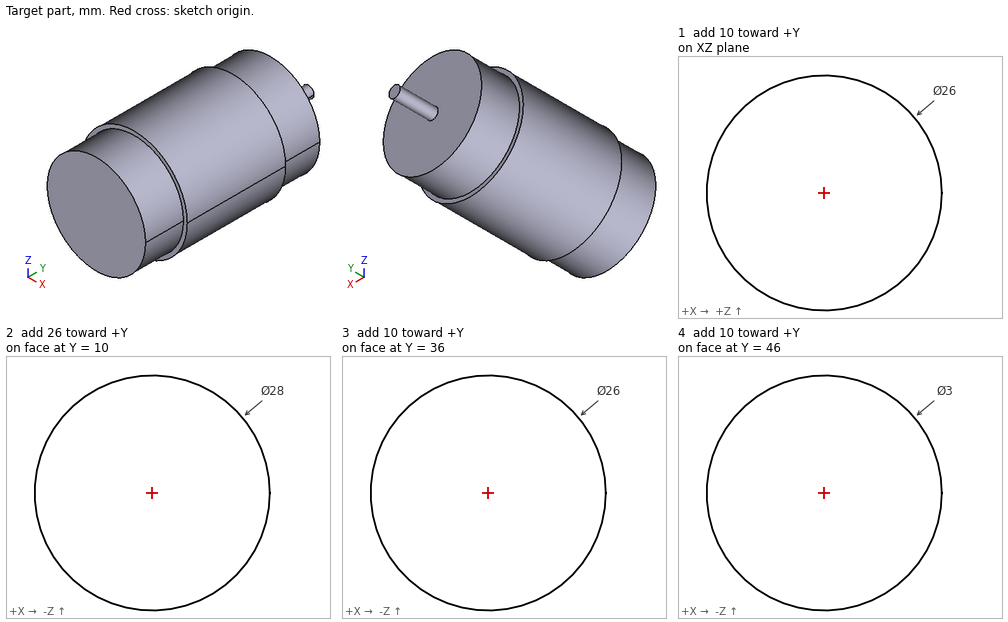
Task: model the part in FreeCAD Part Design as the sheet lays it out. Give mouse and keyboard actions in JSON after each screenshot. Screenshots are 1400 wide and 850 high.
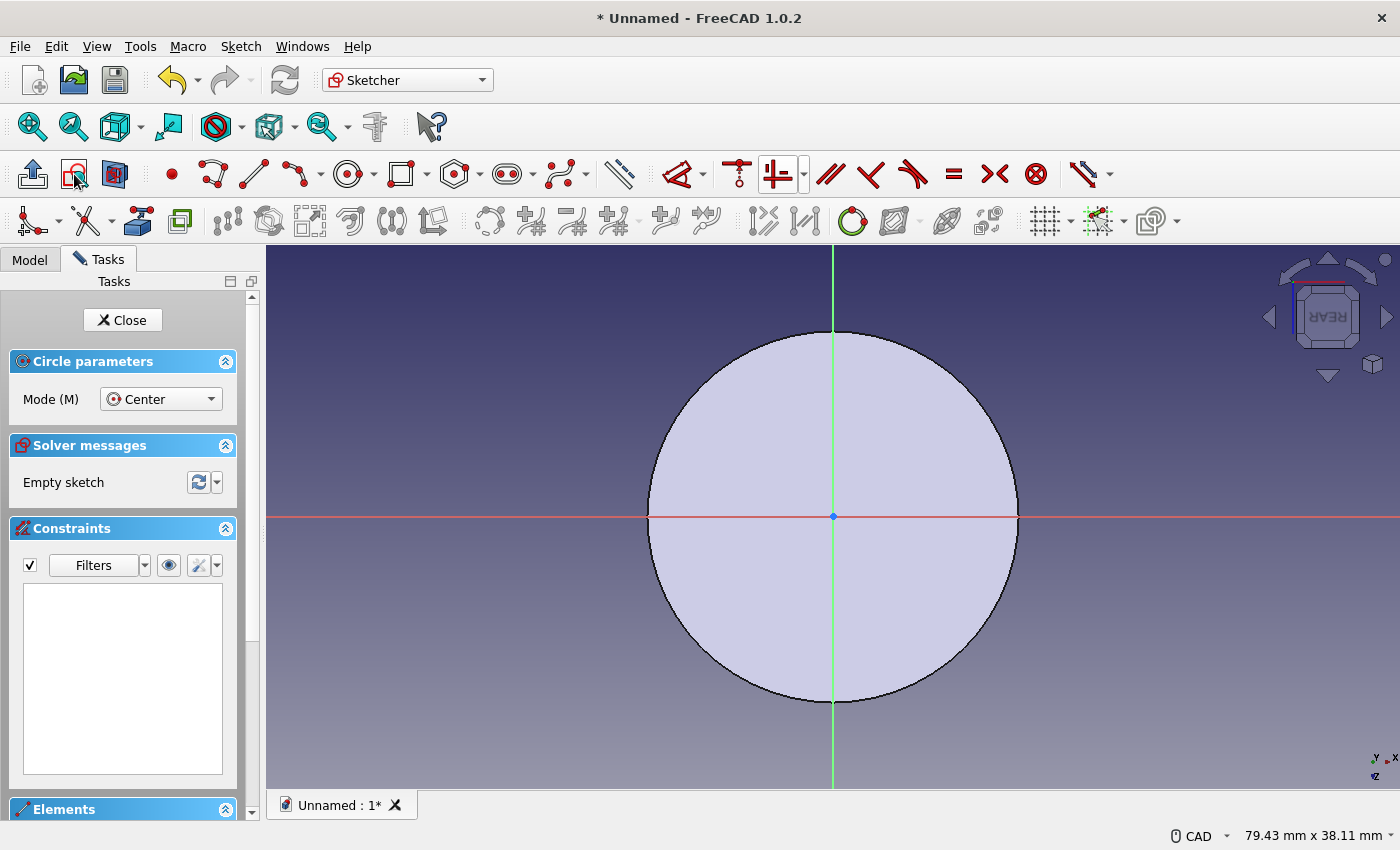
{"action": "left_click", "coordinate": [833, 517]}
{"action": "mouse_move", "coordinate": [974, 376]}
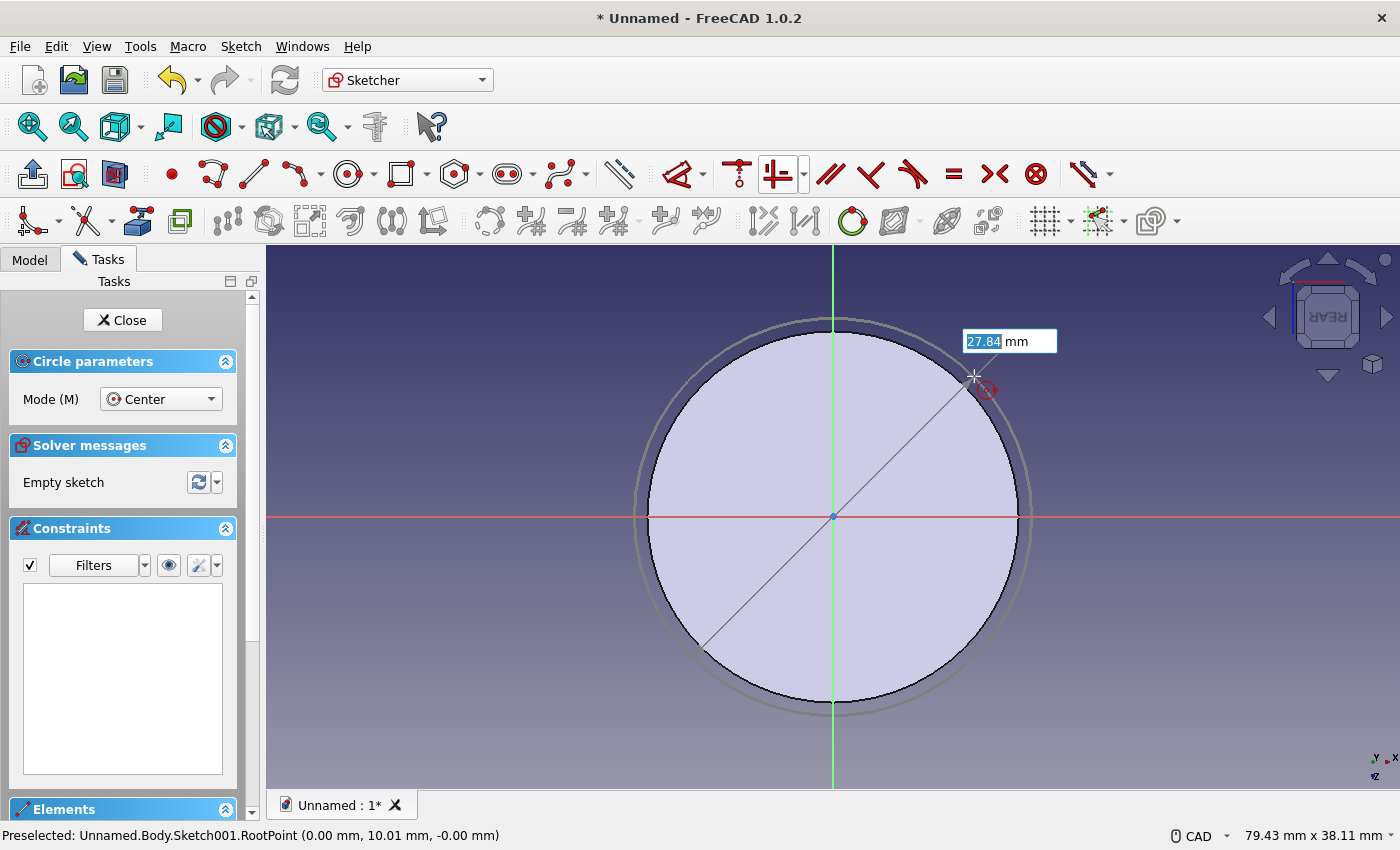
{"action": "type", "text": "28"}
{"action": "key", "text": "Return"}
{"action": "key", "text": "Escape"}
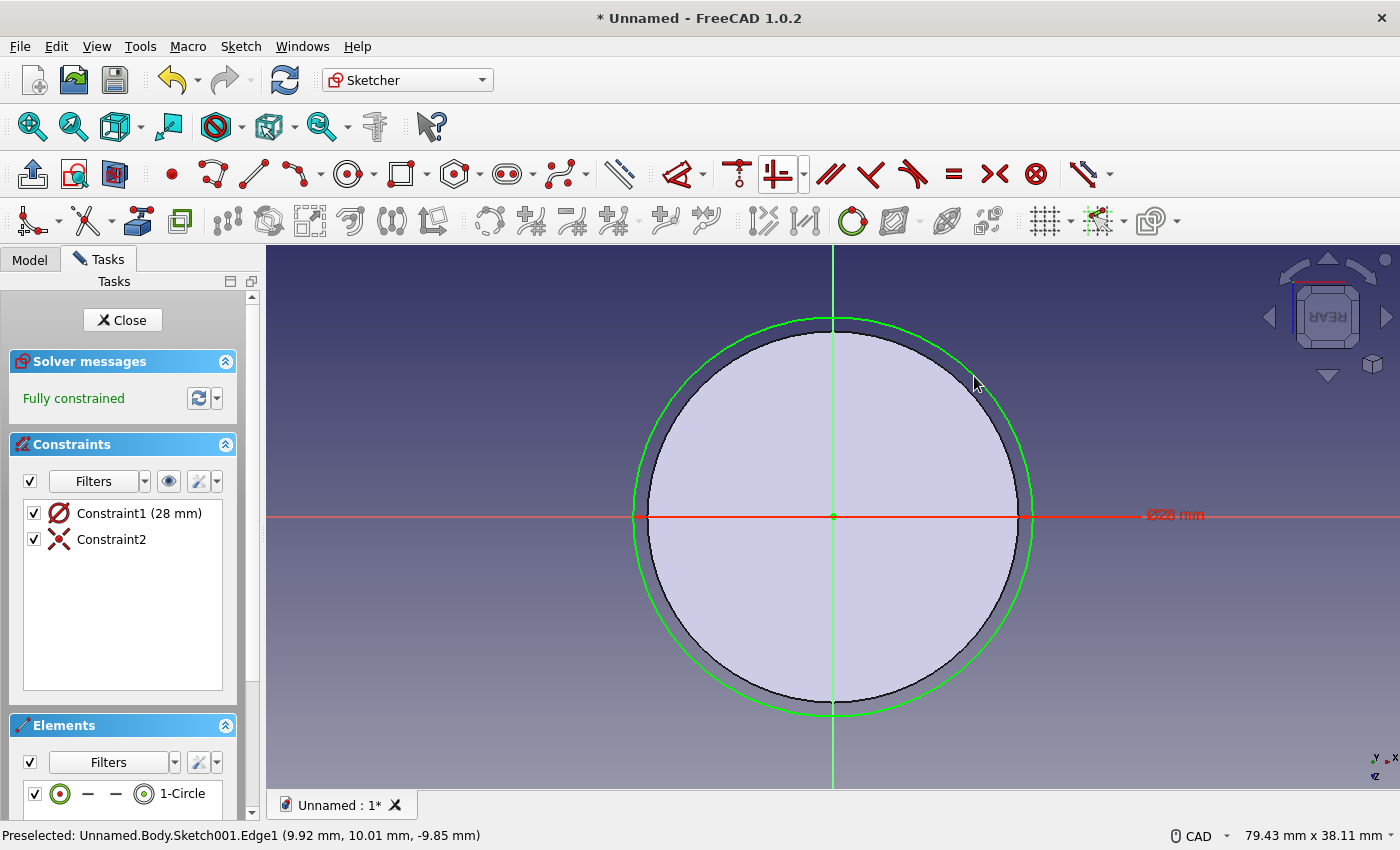
{"action": "left_click", "coordinate": [123, 320]}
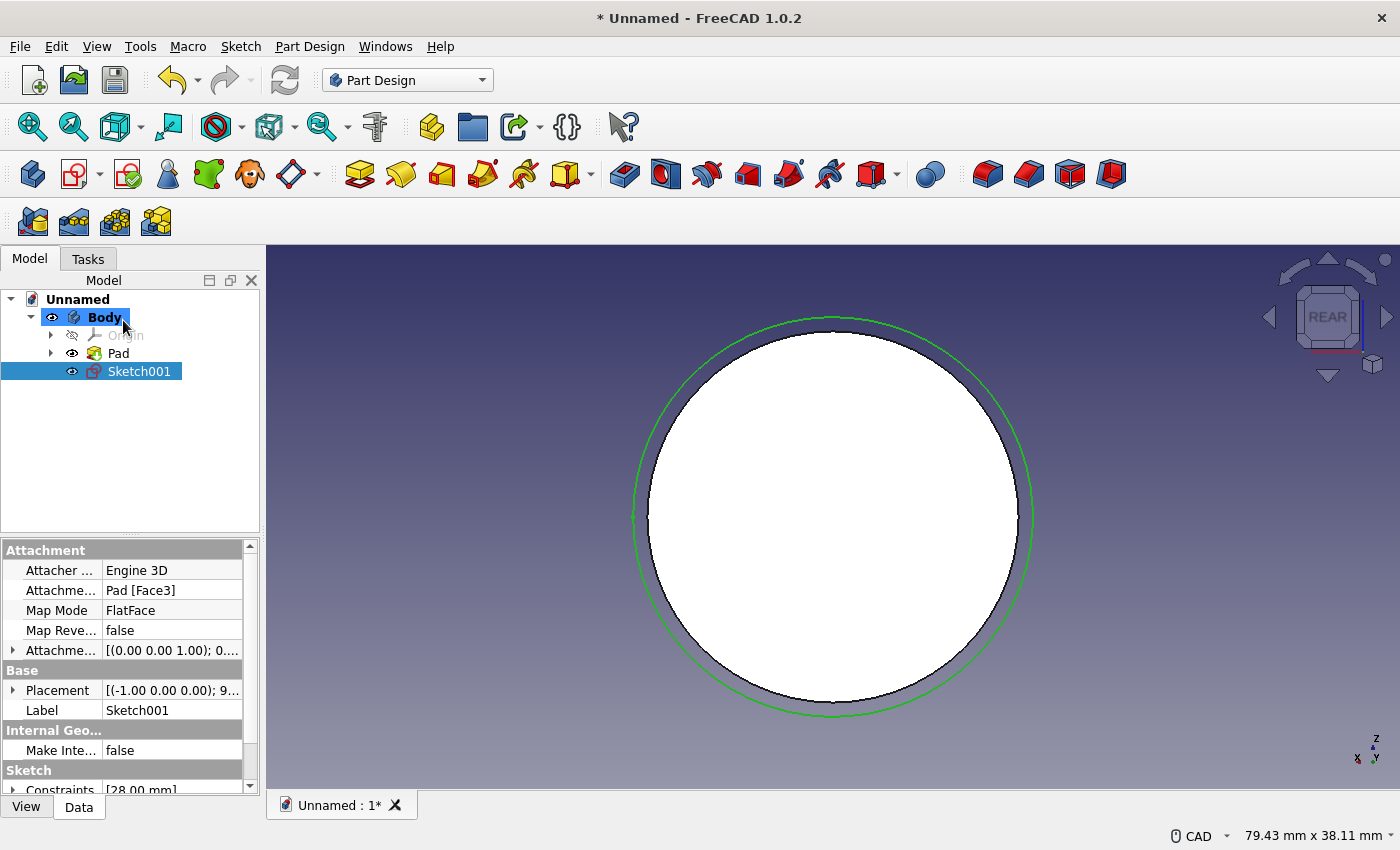
{"action": "left_click", "coordinate": [360, 174]}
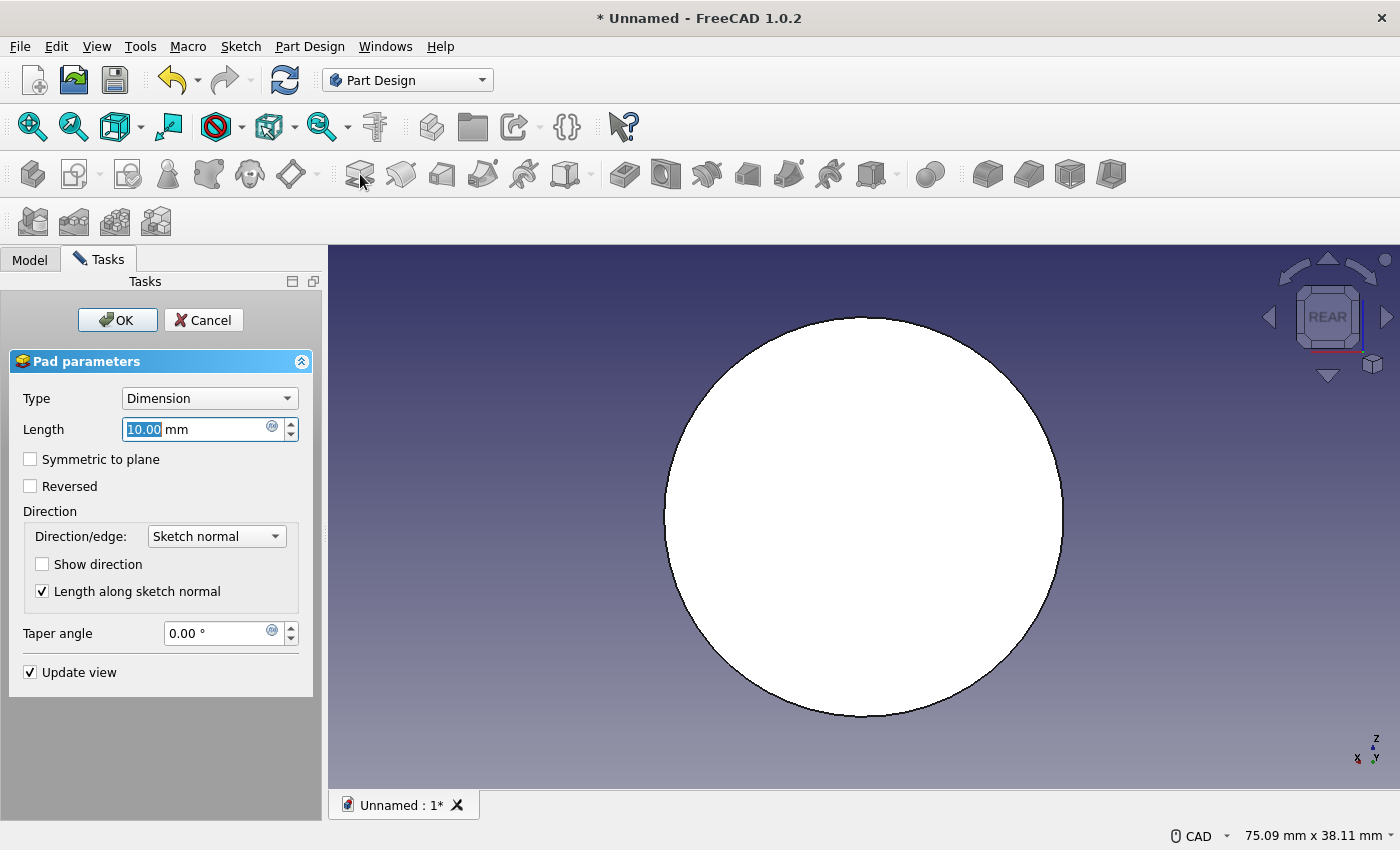
{"action": "type", "text": "26"}
{"action": "key", "text": "Tab"}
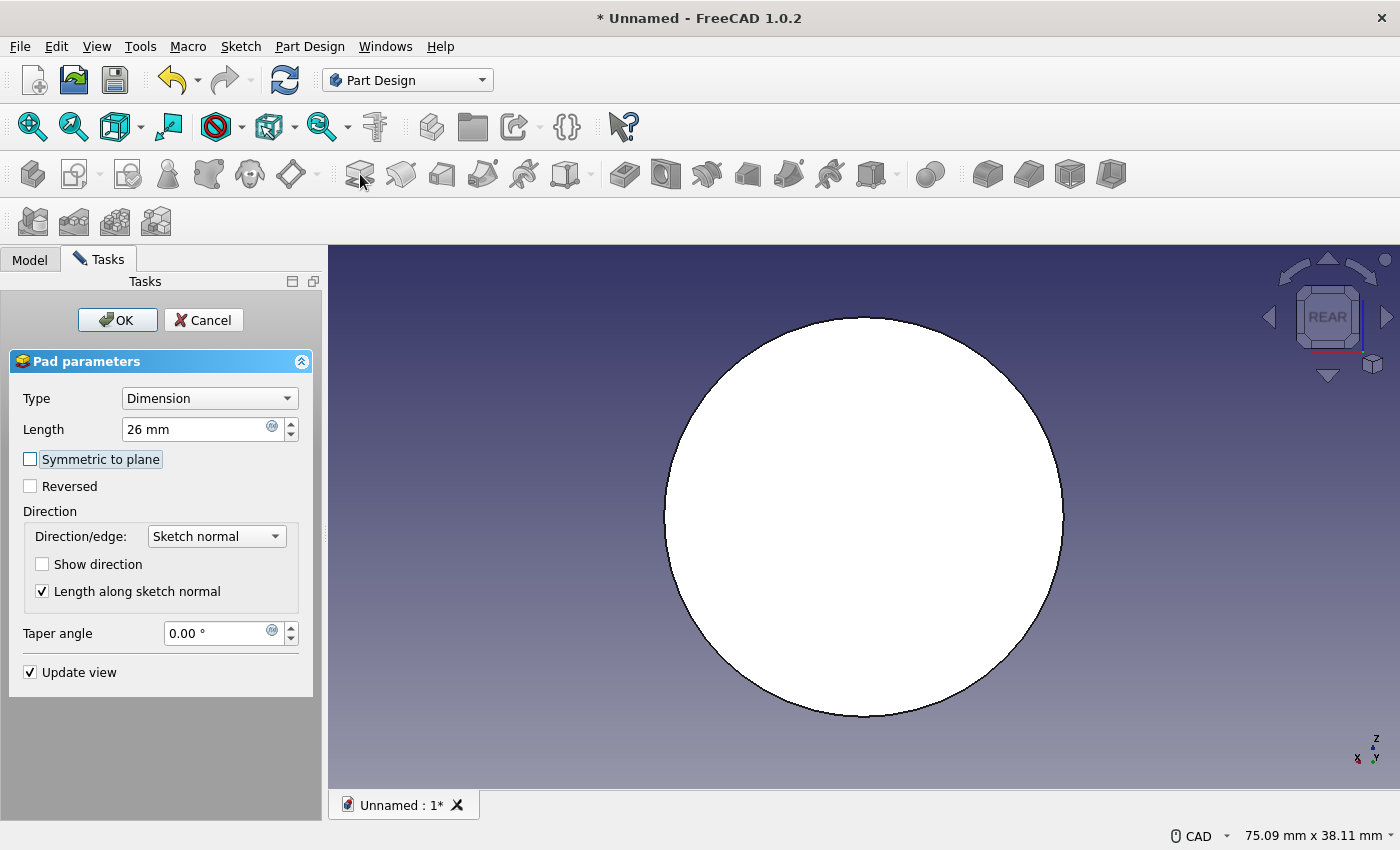
{"action": "left_click", "coordinate": [118, 320]}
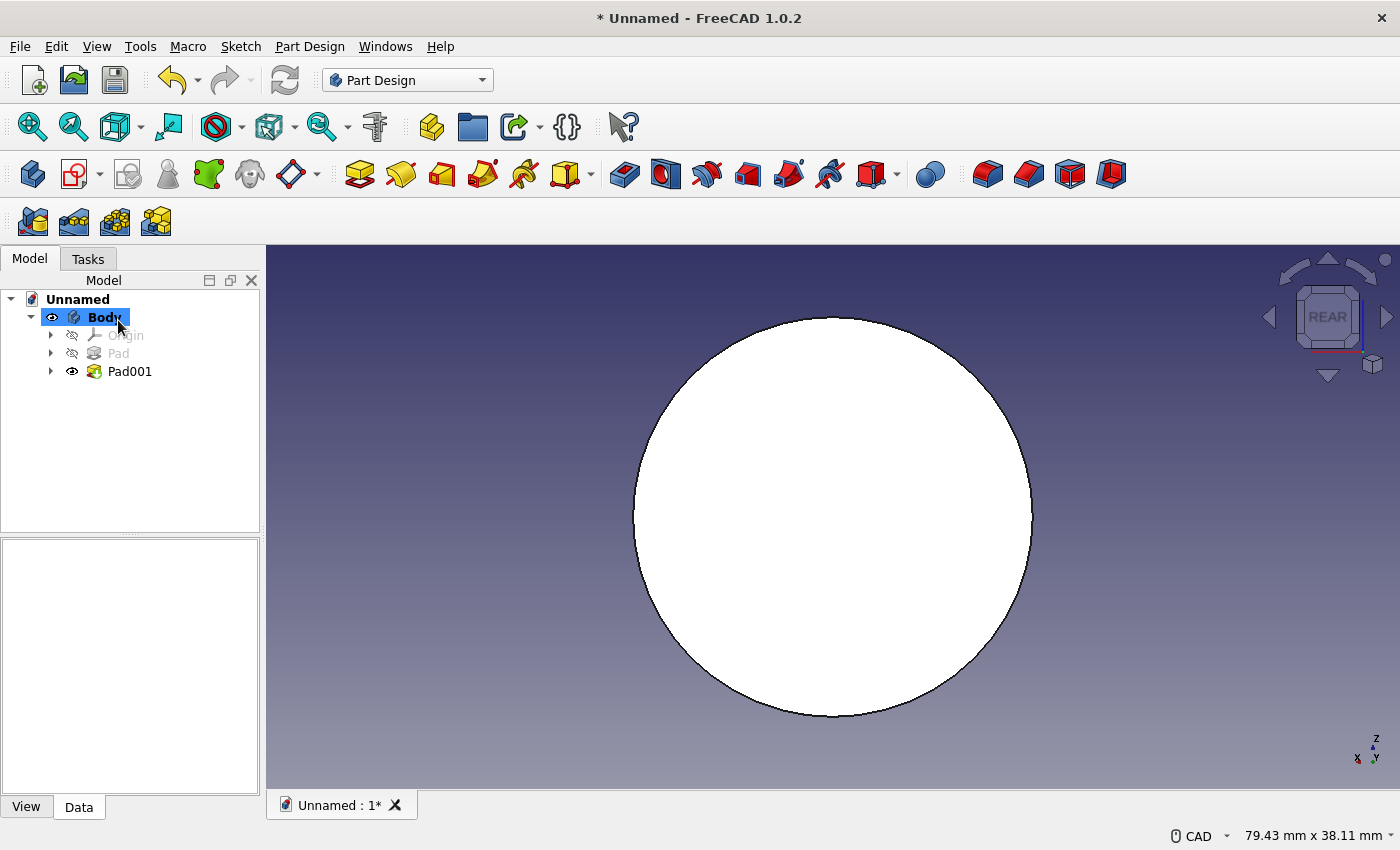
{"action": "left_click", "coordinate": [833, 516]}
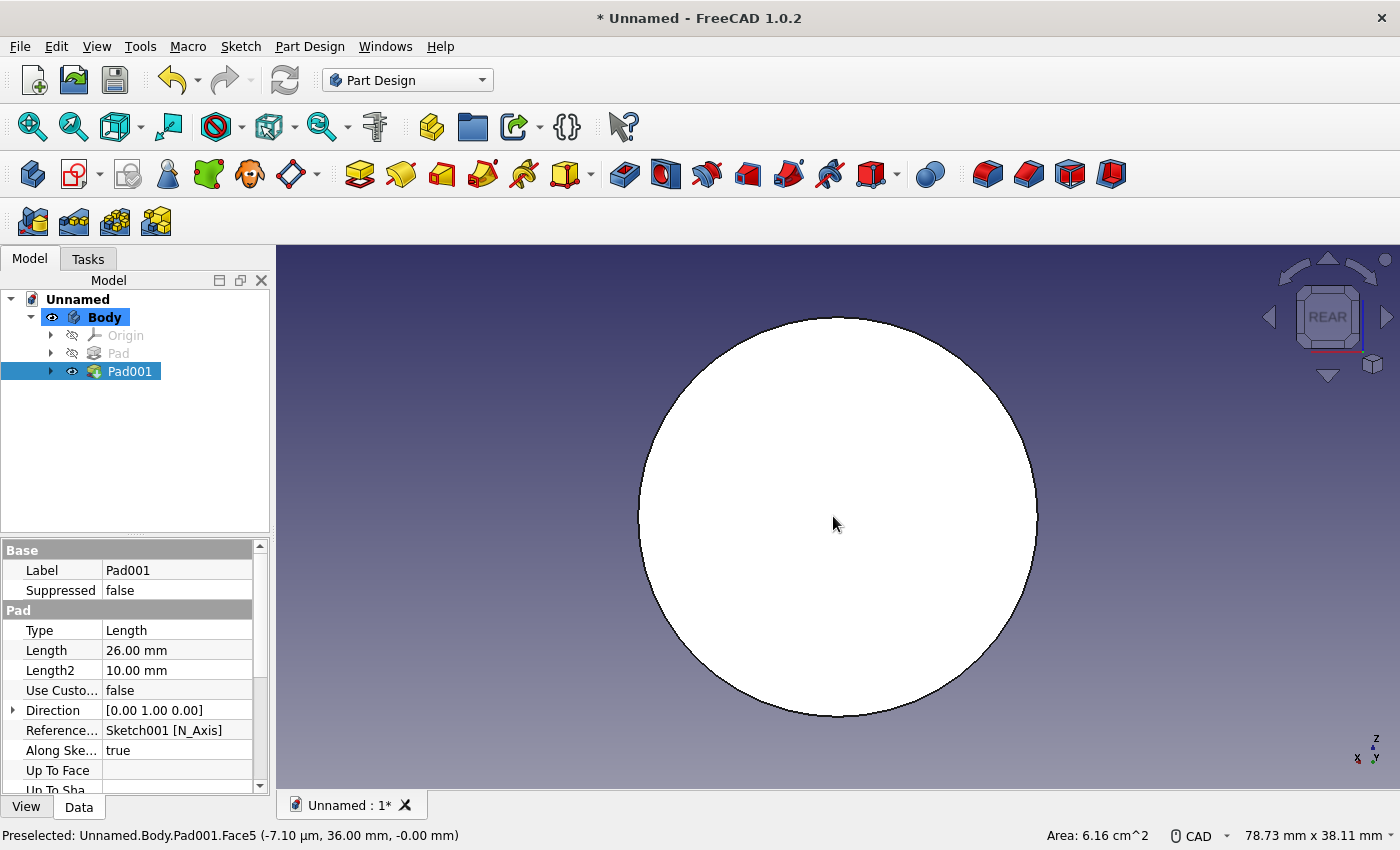
{"action": "left_click", "coordinate": [74, 174]}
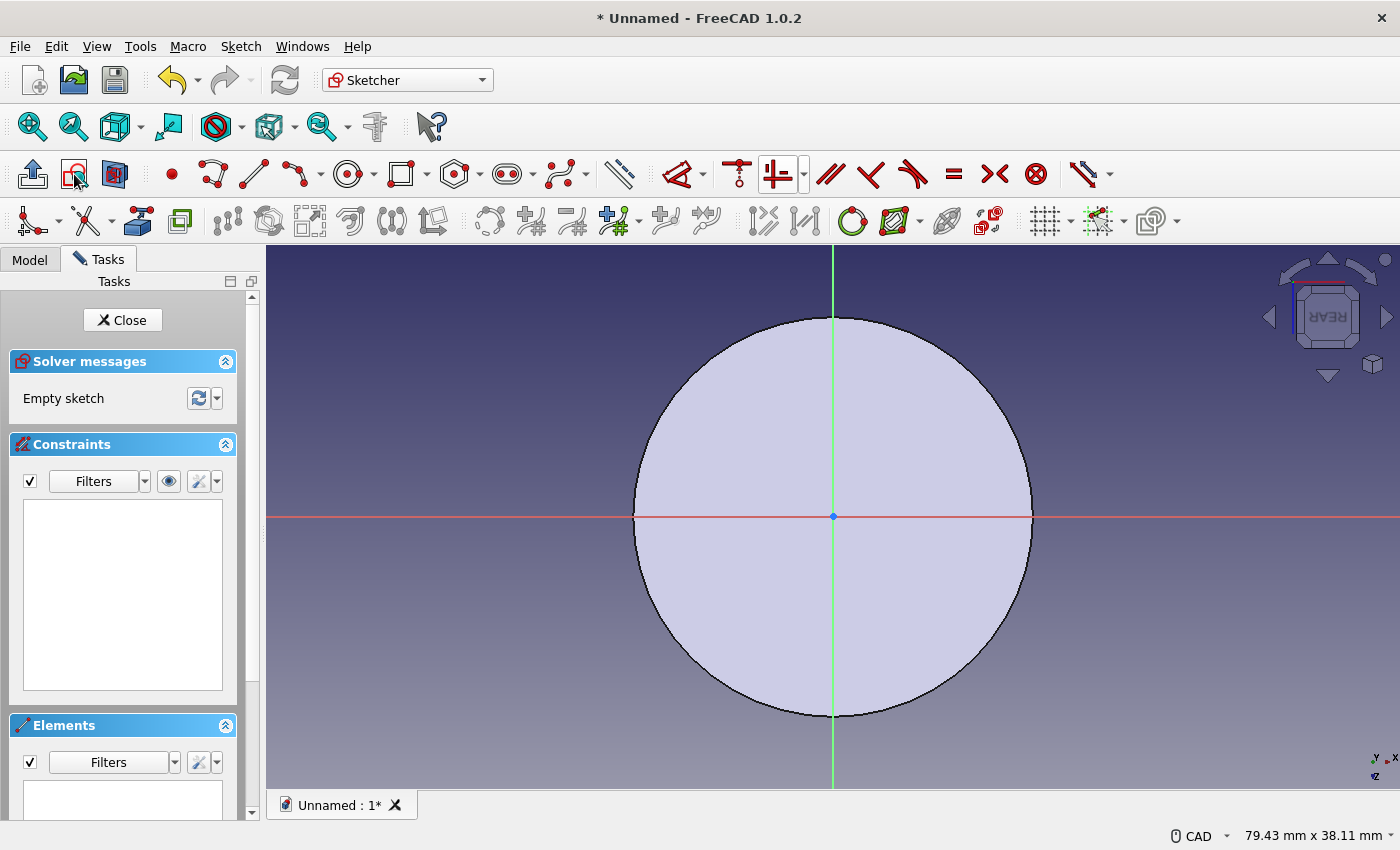
{"action": "left_click", "coordinate": [348, 174]}